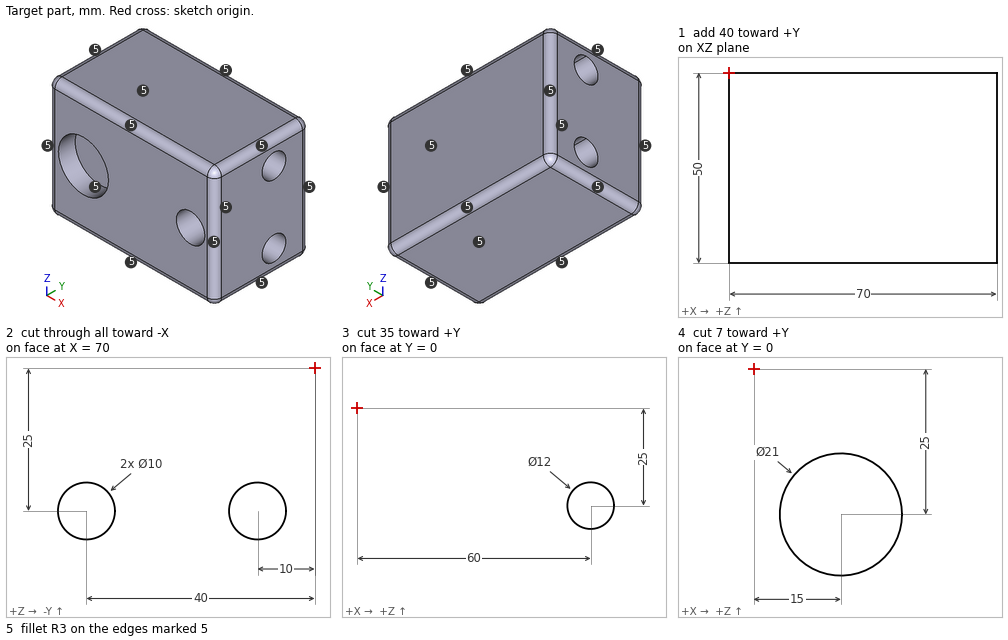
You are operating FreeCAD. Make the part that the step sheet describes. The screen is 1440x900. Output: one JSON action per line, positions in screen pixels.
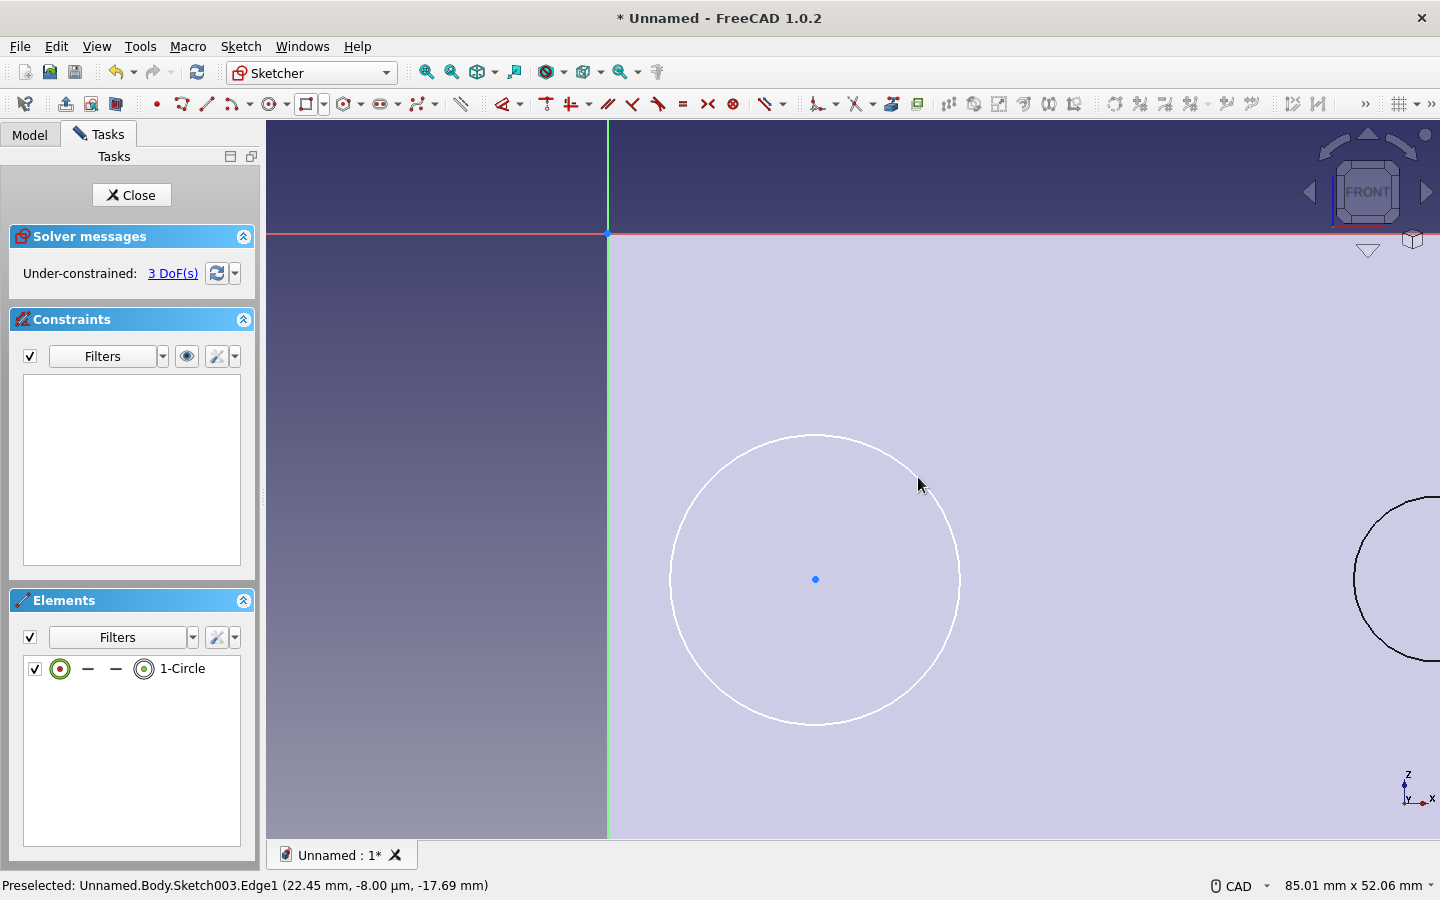
{"action": "left_click", "coordinate": [917, 477]}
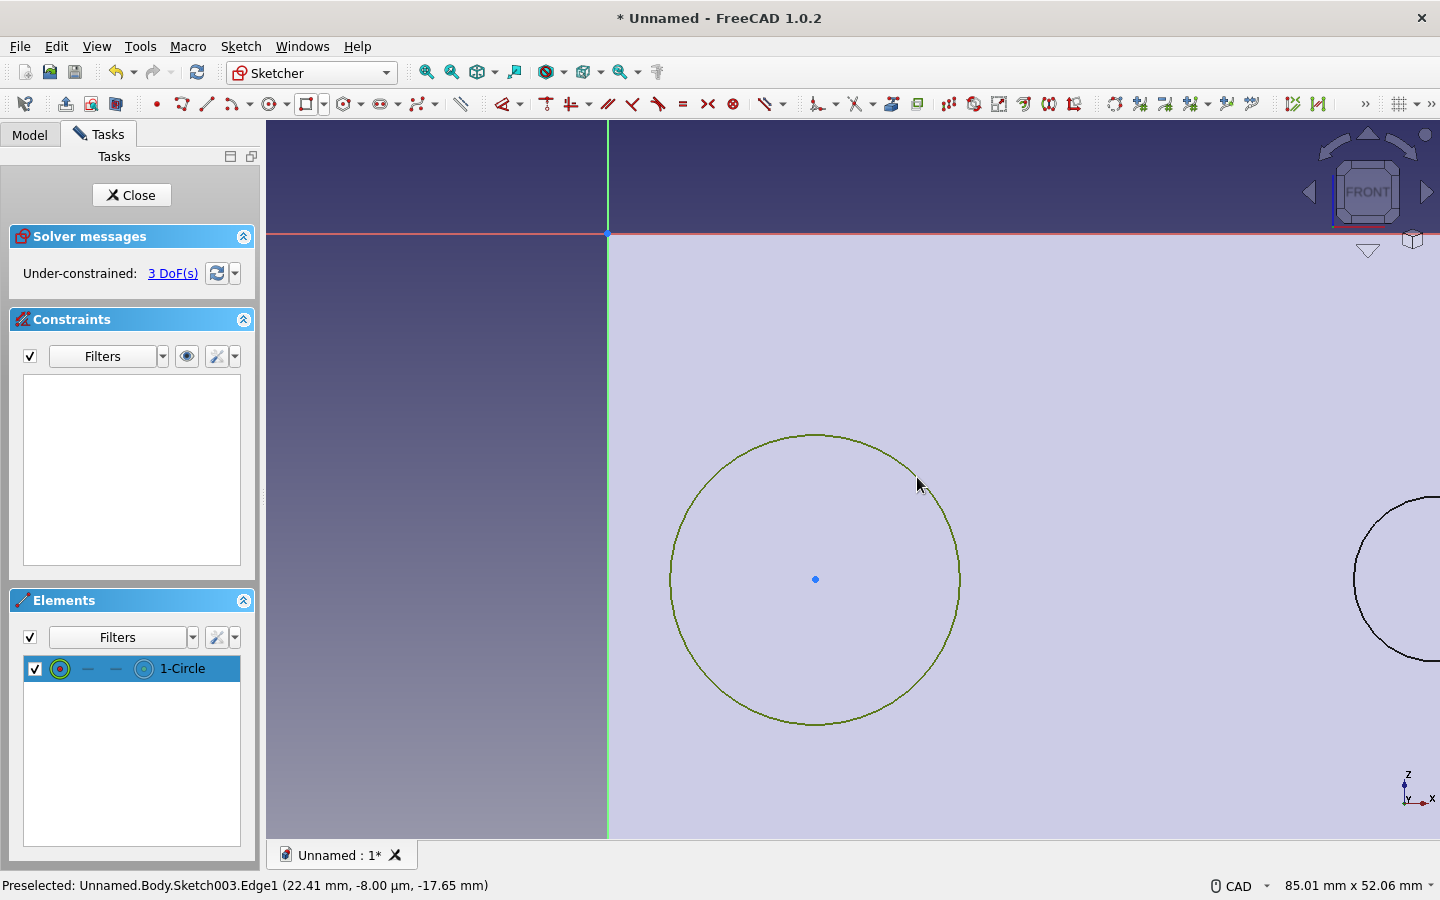
{"action": "key", "text": "k o"}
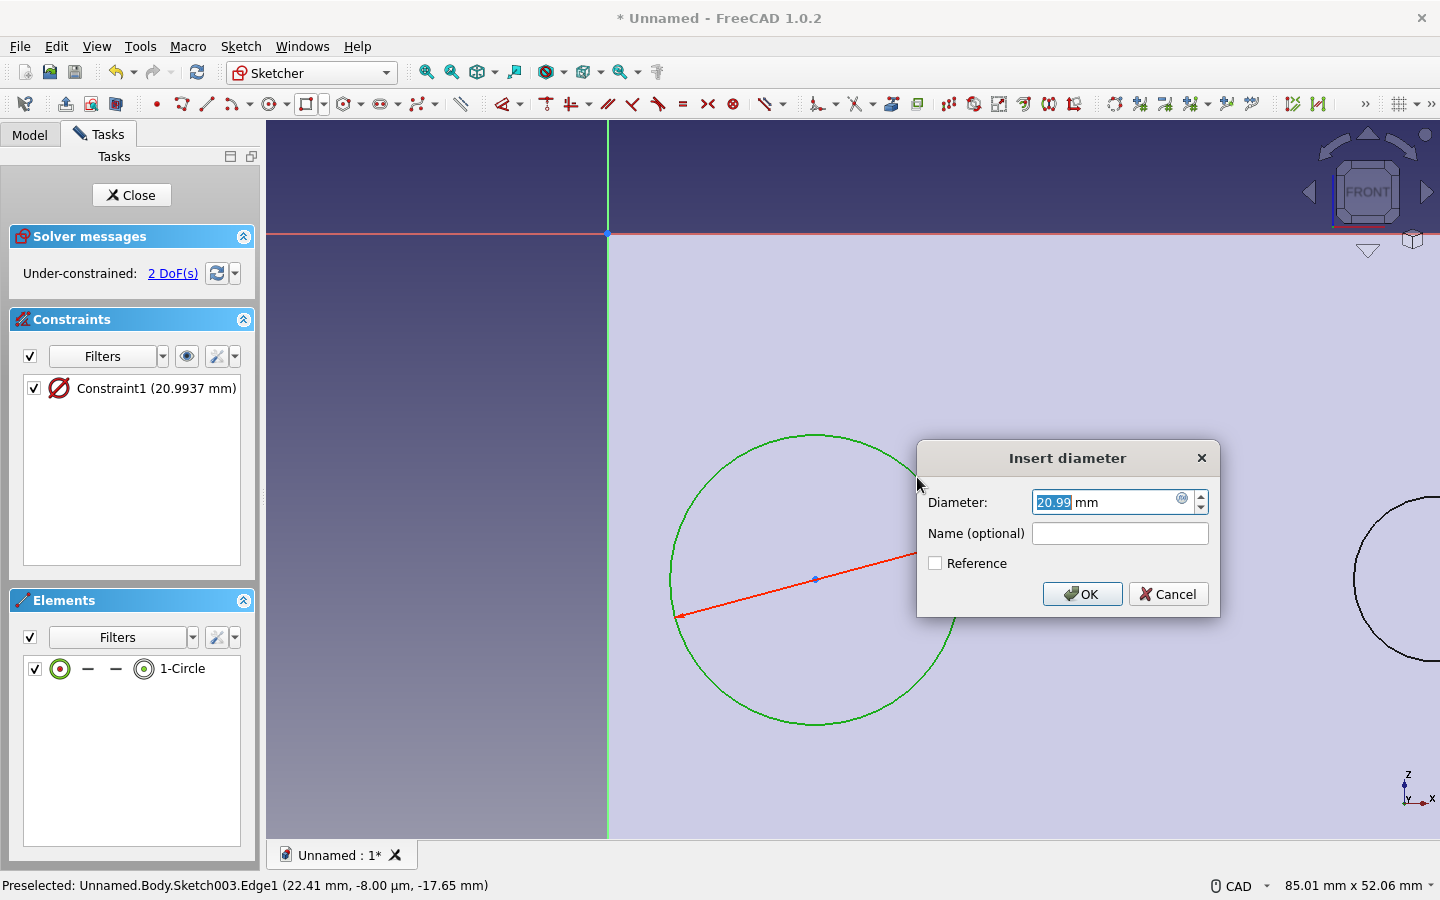
{"action": "type", "text": "21"}
{"action": "key", "text": "Return"}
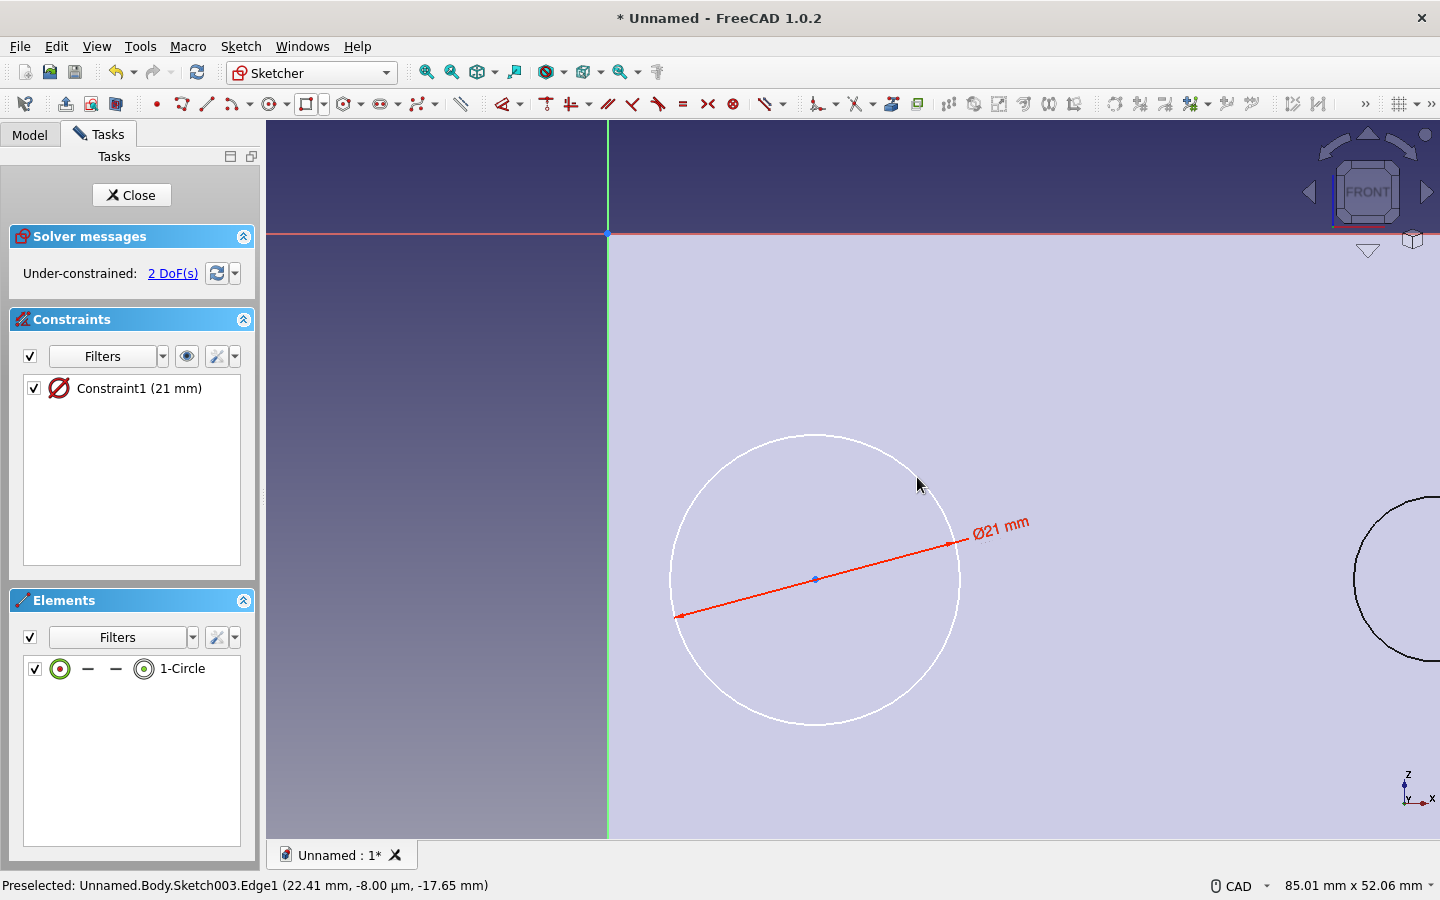
{"action": "left_click", "coordinate": [815, 580]}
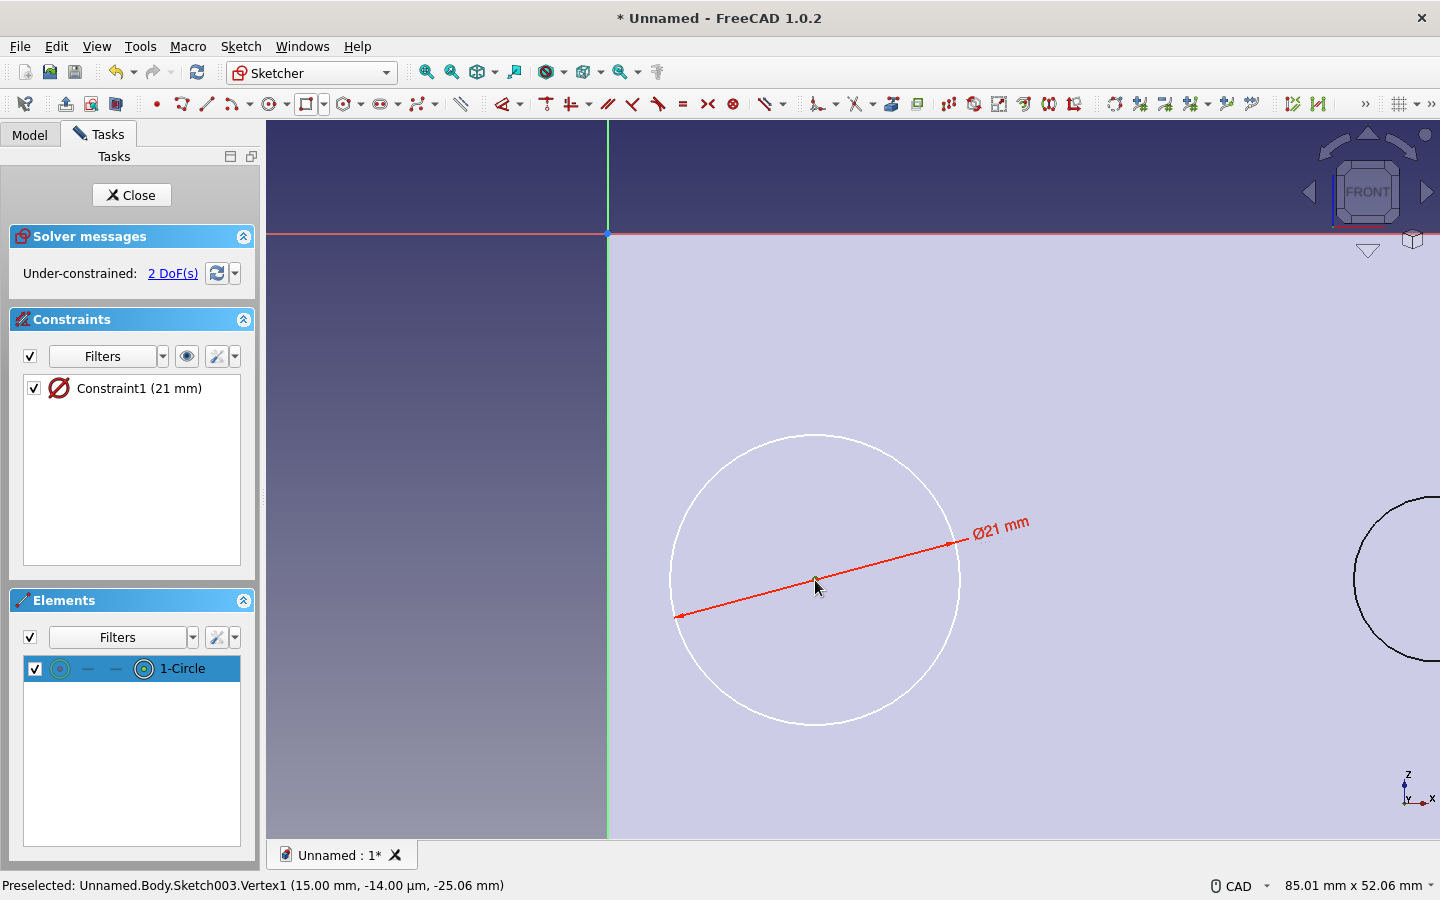
{"action": "left_click", "coordinate": [520, 104]}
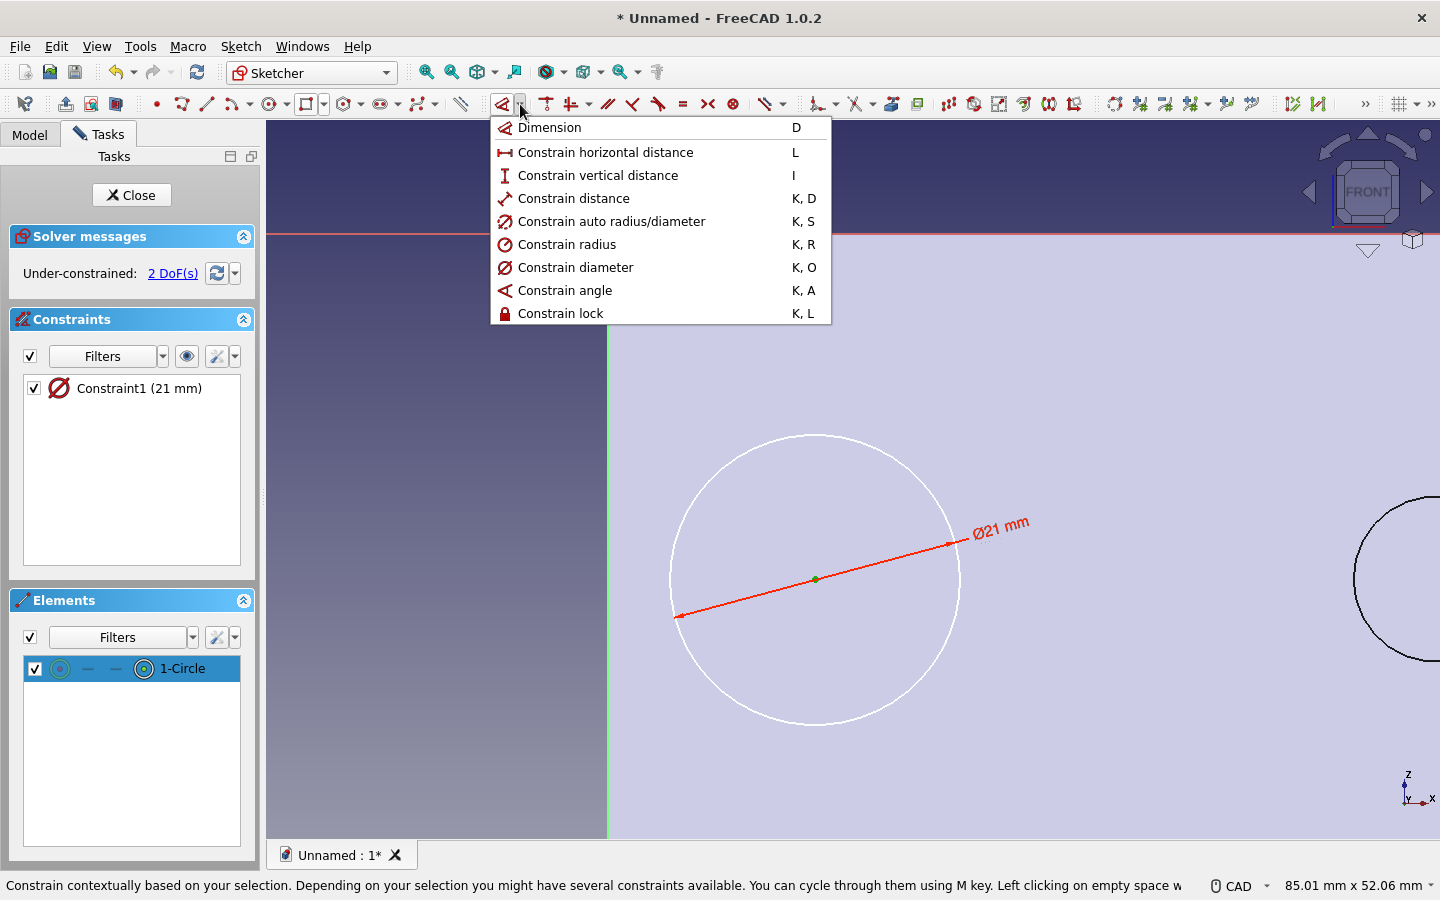
{"action": "left_click", "coordinate": [661, 152]}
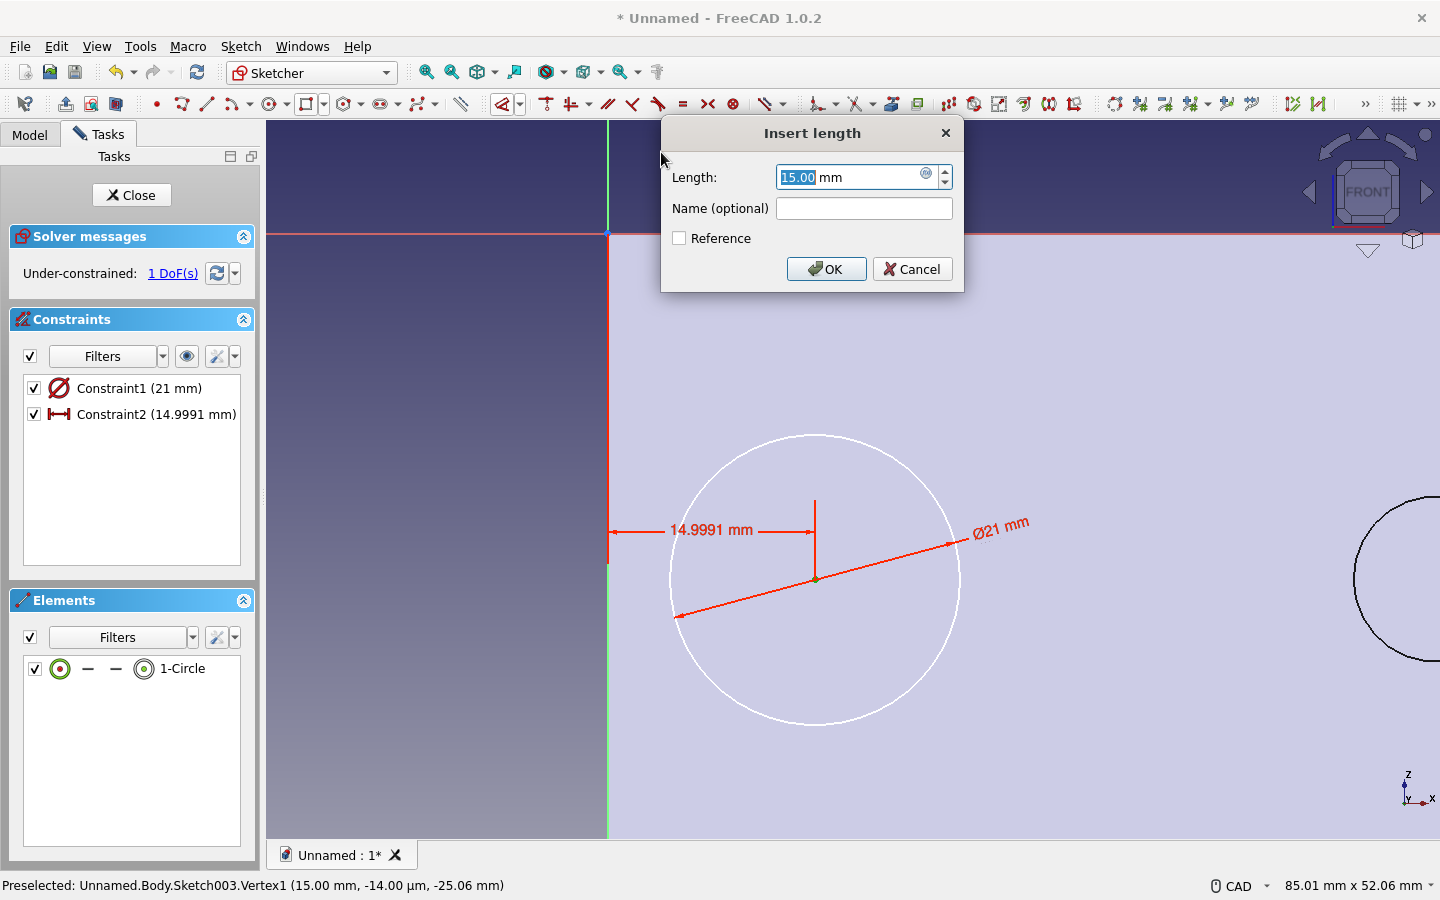
{"action": "type", "text": "15"}
{"action": "key", "text": "Return"}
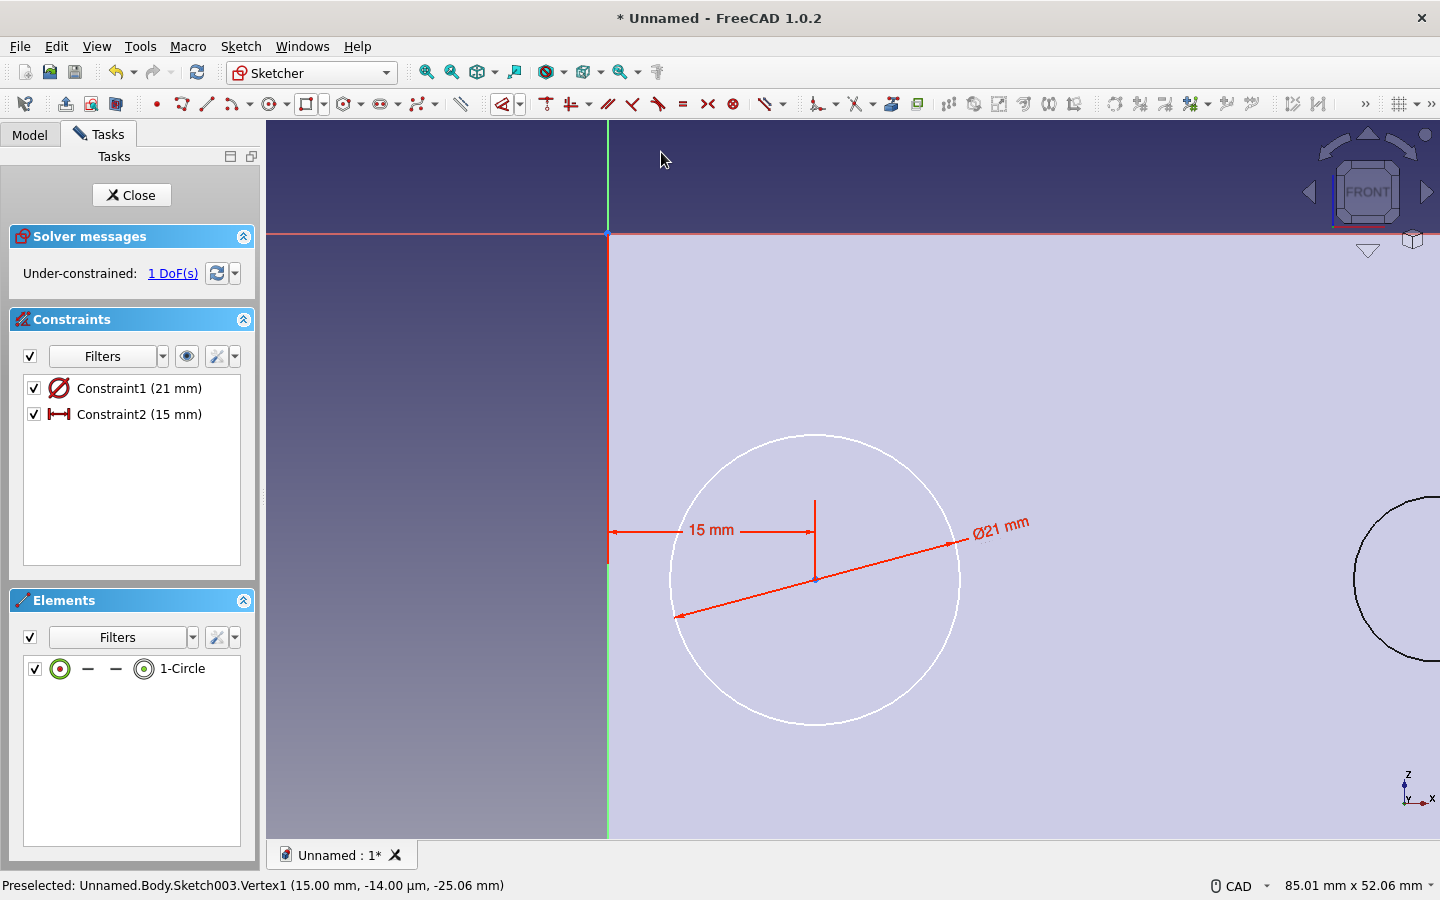
{"action": "left_click", "coordinate": [815, 580]}